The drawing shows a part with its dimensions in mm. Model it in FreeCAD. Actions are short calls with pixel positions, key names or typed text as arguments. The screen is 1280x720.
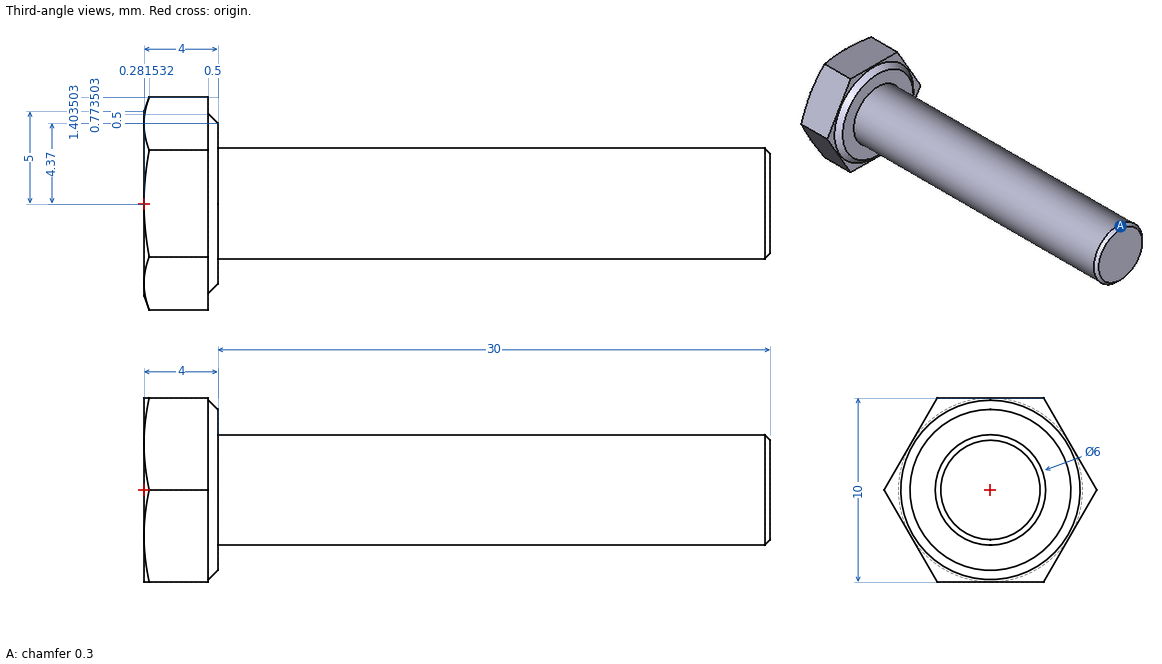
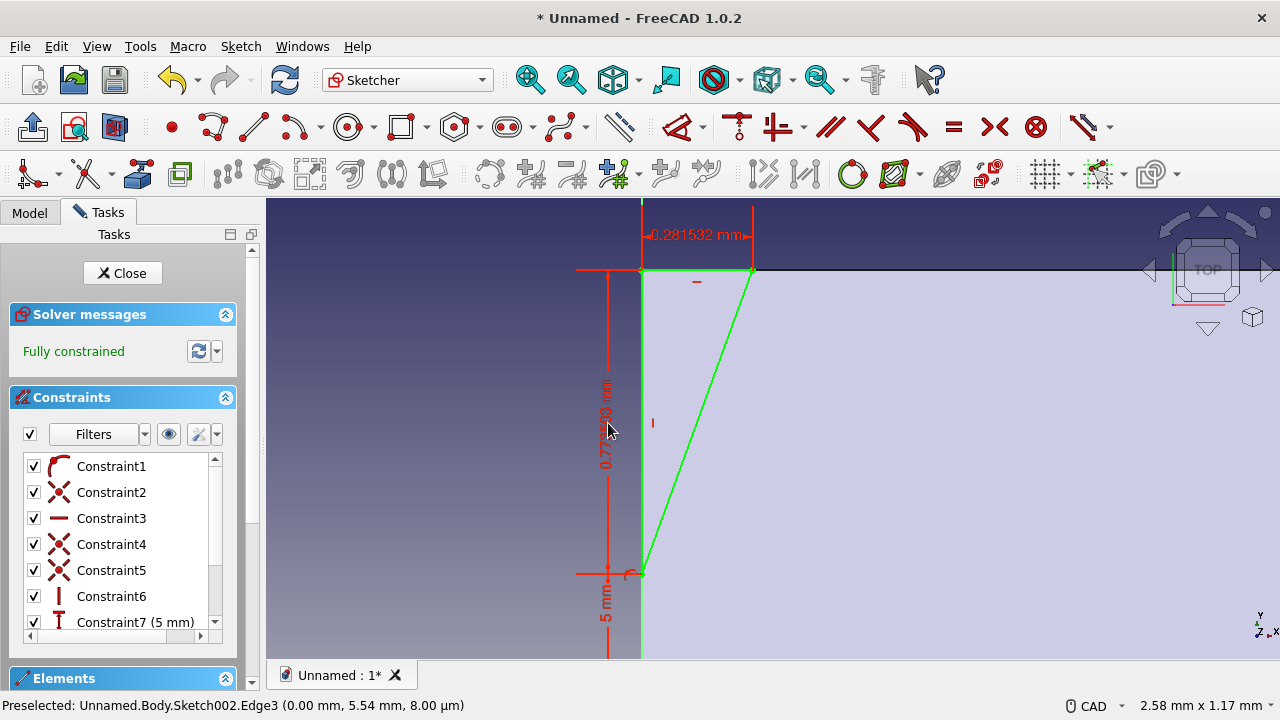
click(123, 273)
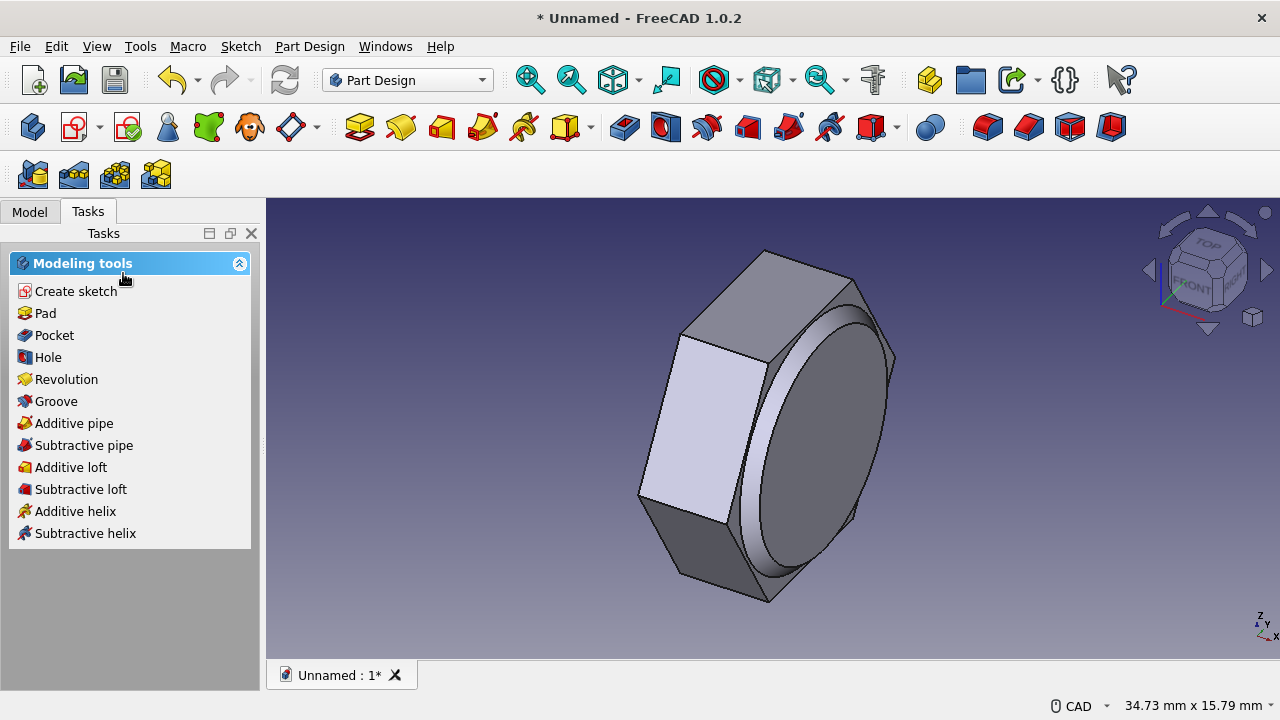
click(707, 128)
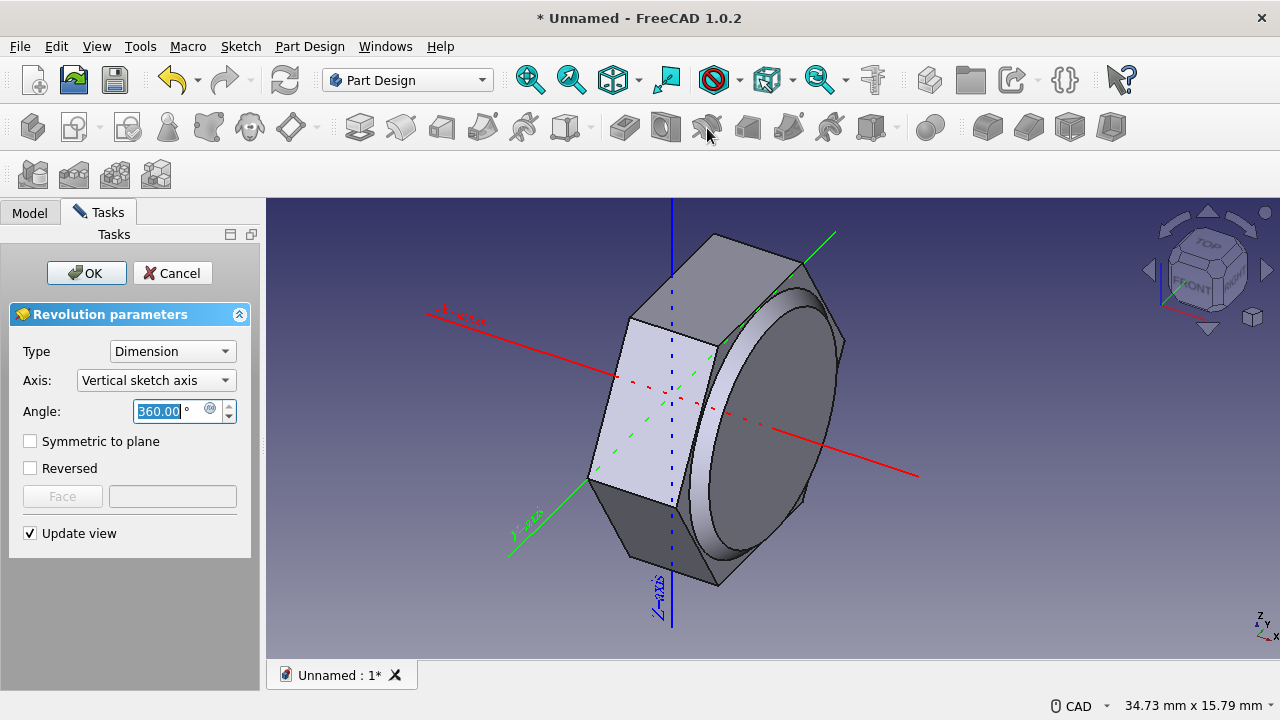
click(157, 380)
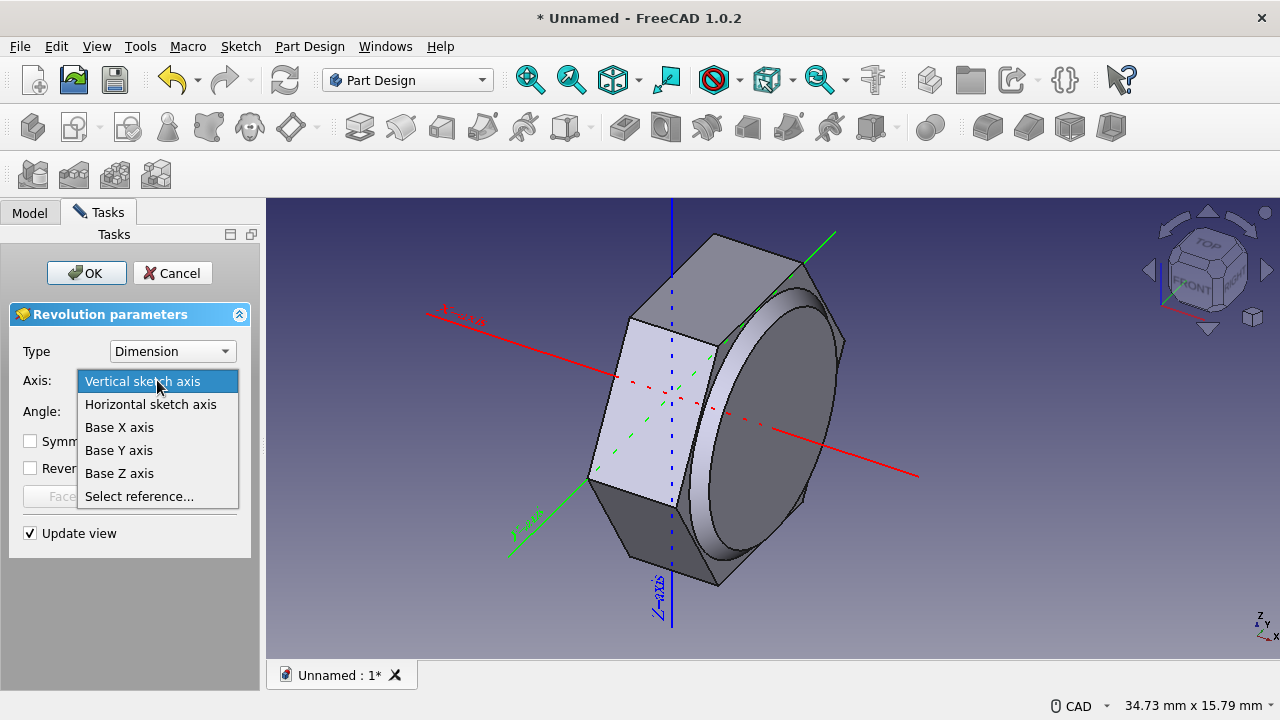
click(156, 404)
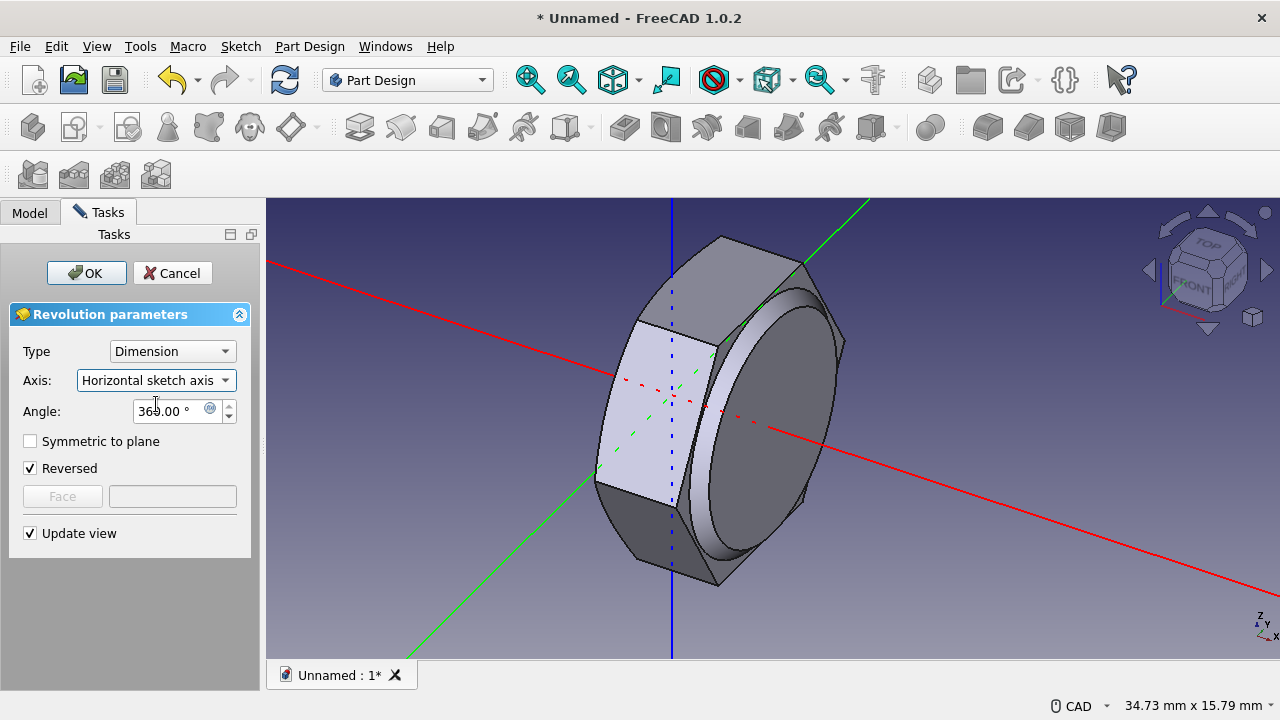
click(87, 273)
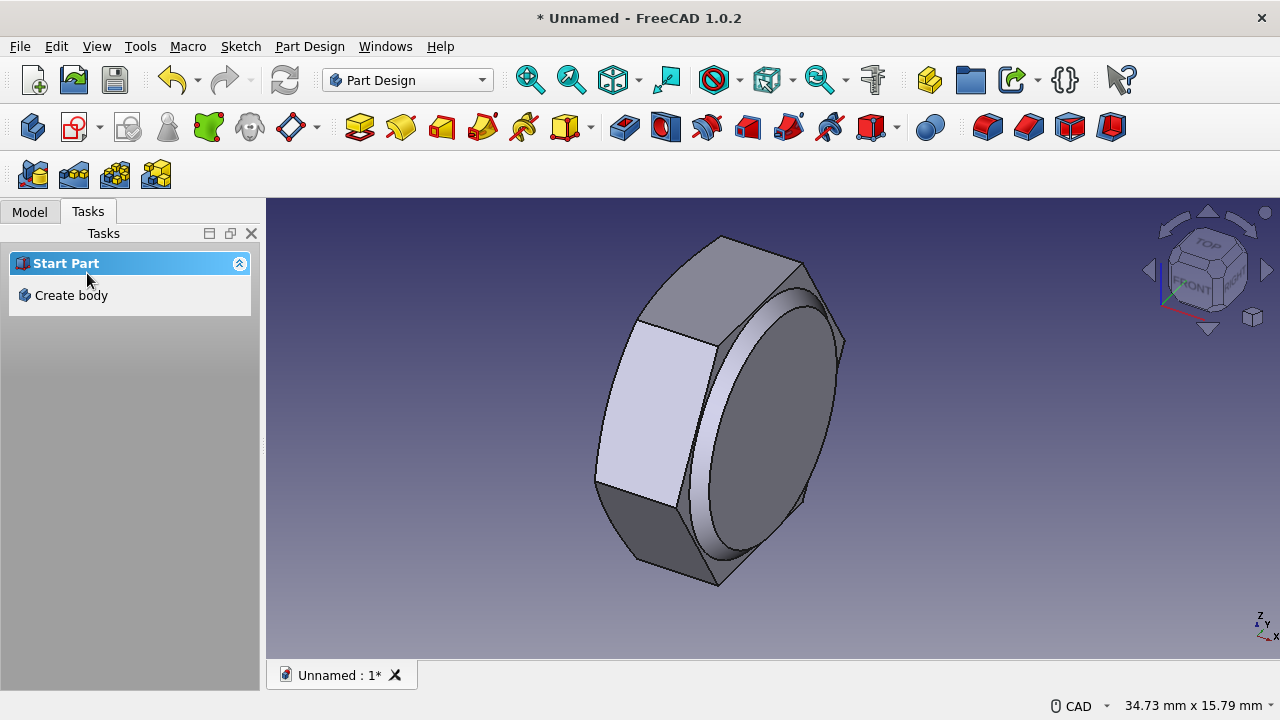
click(531, 80)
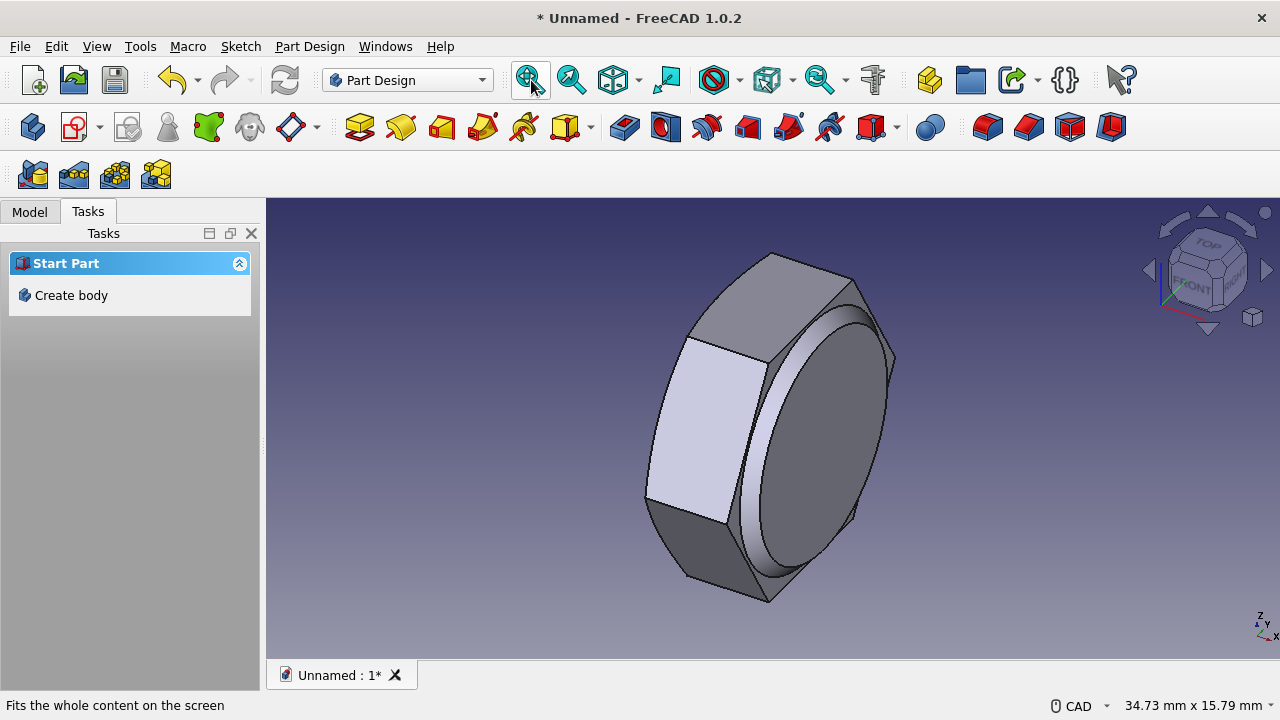
click(824, 444)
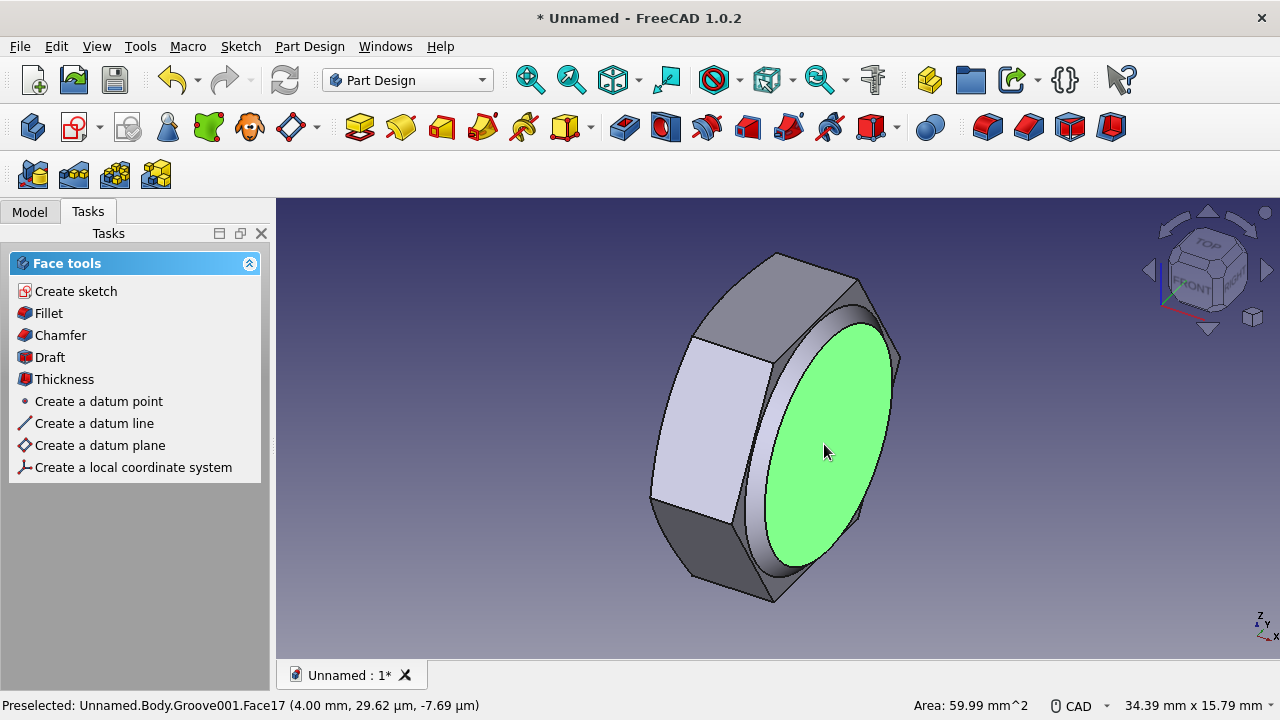
click(74, 128)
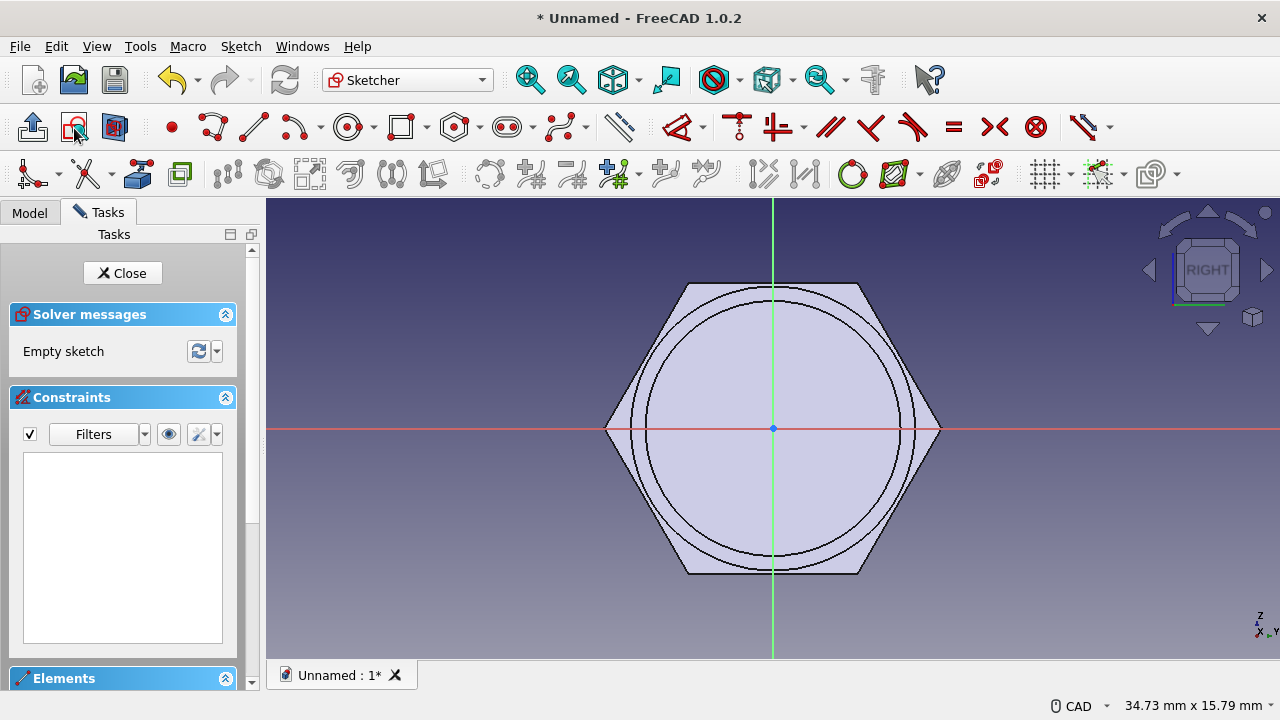
scroll(912, 428, up, 2)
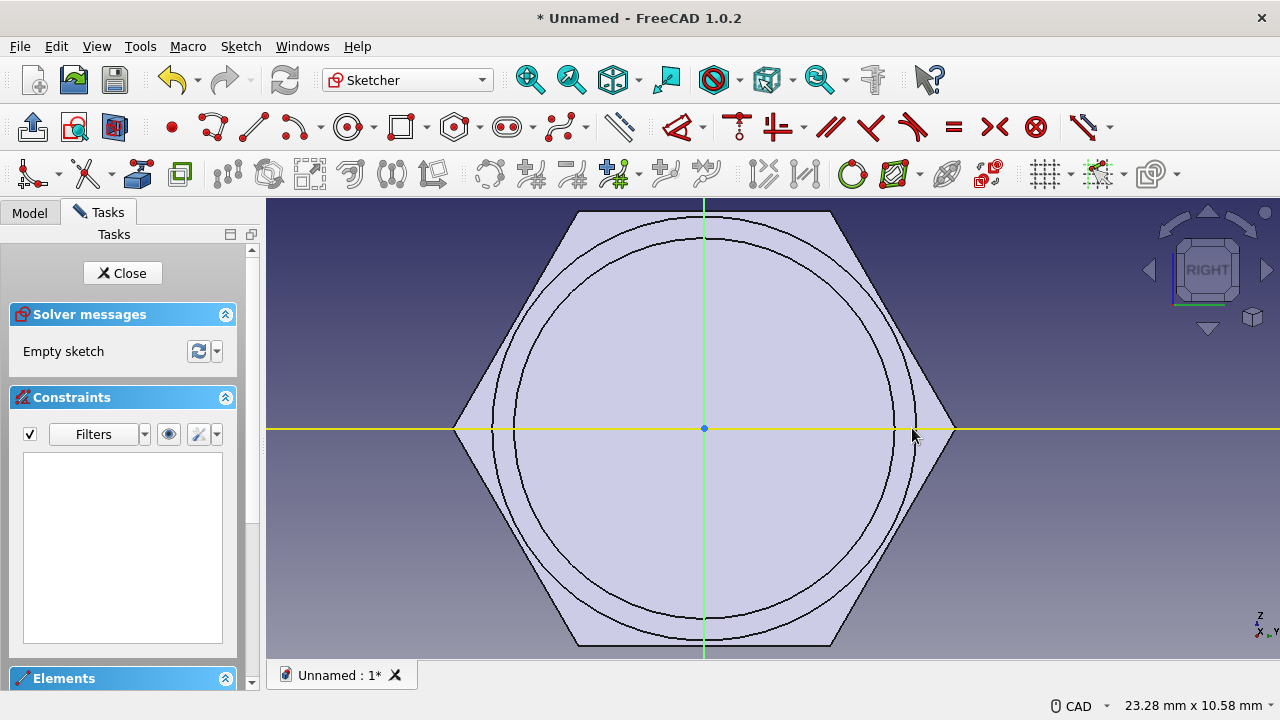
click(348, 128)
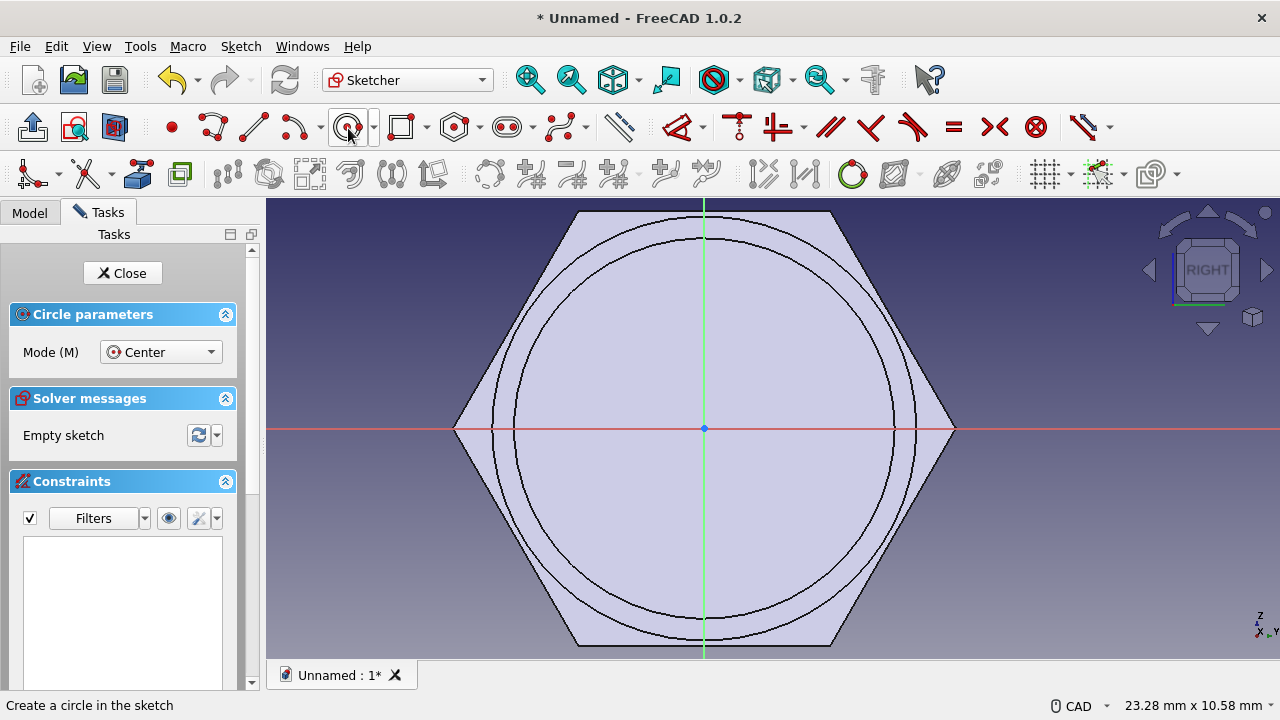
click(704, 428)
move(797, 336)